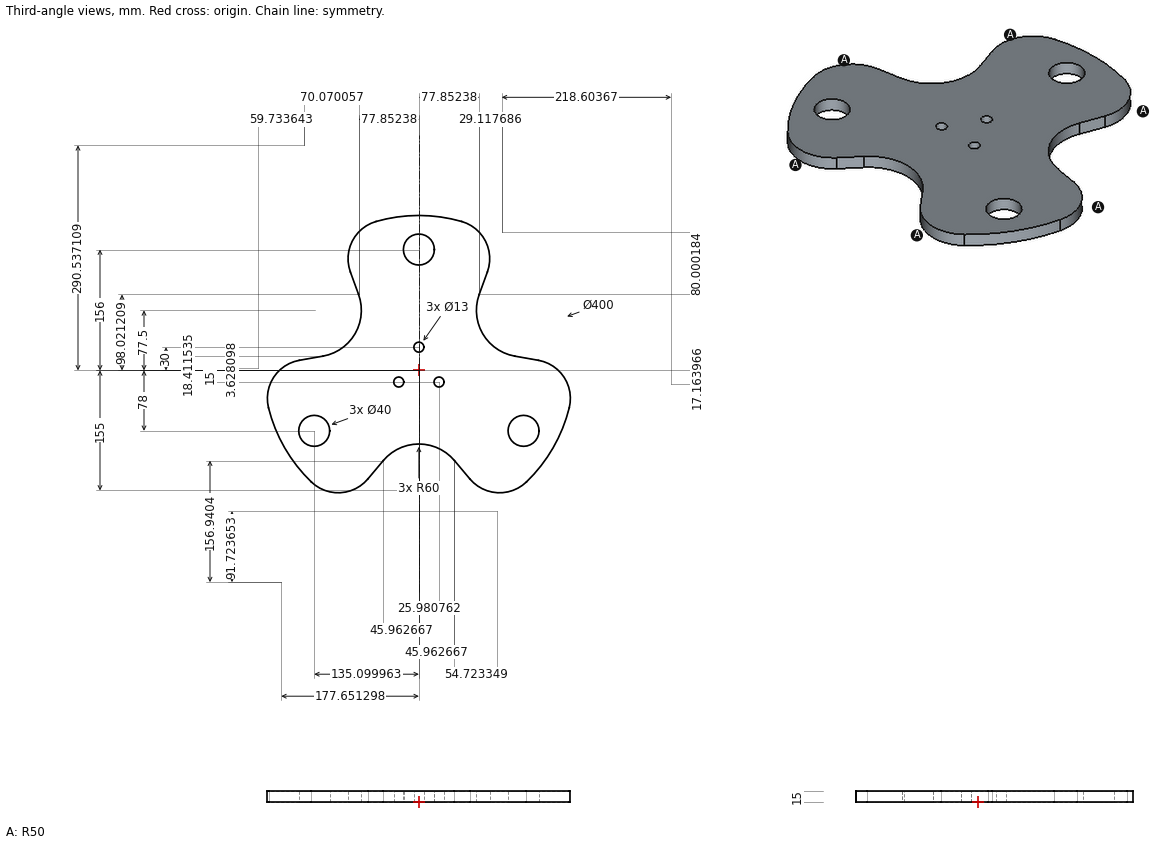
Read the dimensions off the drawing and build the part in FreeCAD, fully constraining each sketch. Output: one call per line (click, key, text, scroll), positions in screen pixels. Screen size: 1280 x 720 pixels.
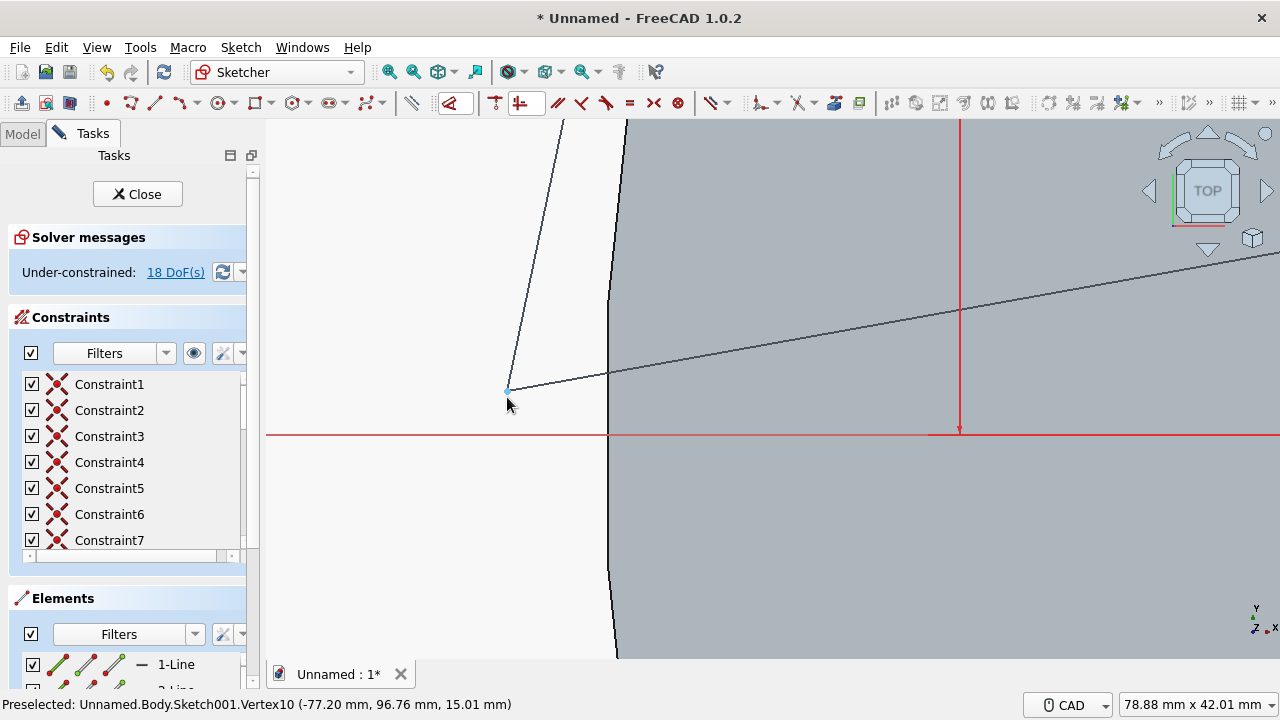
click(507, 391)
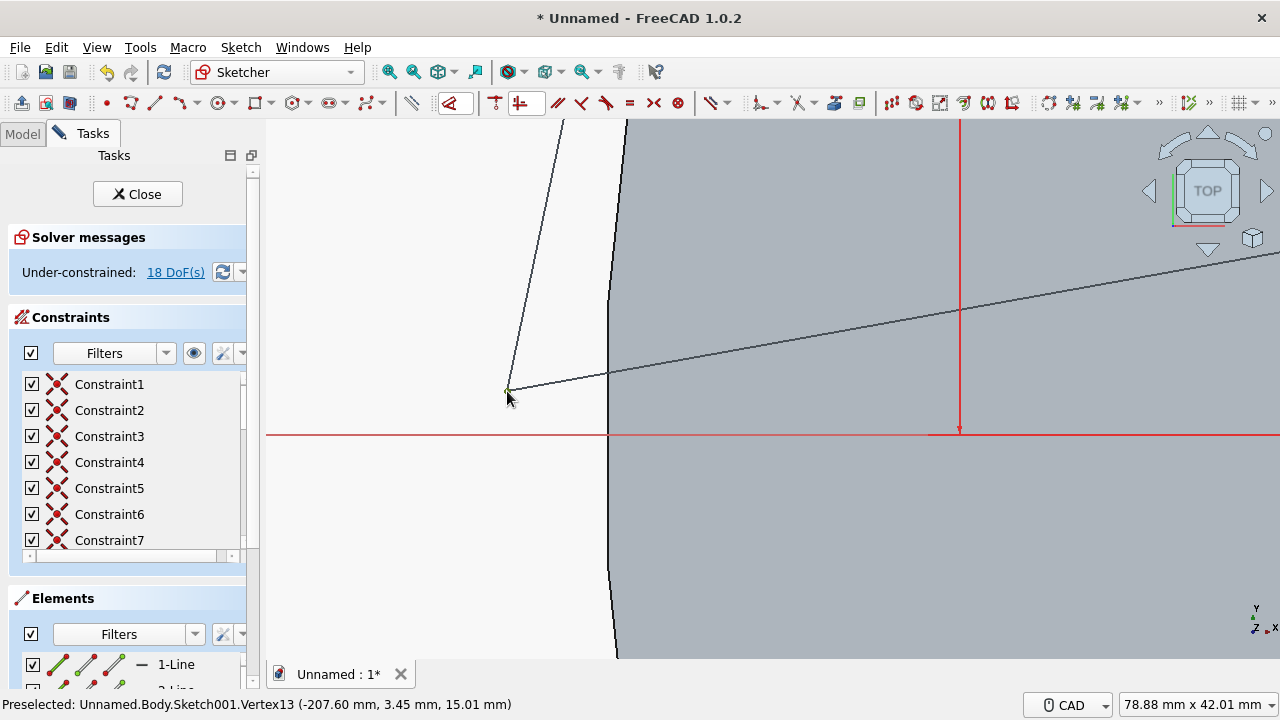
key(i)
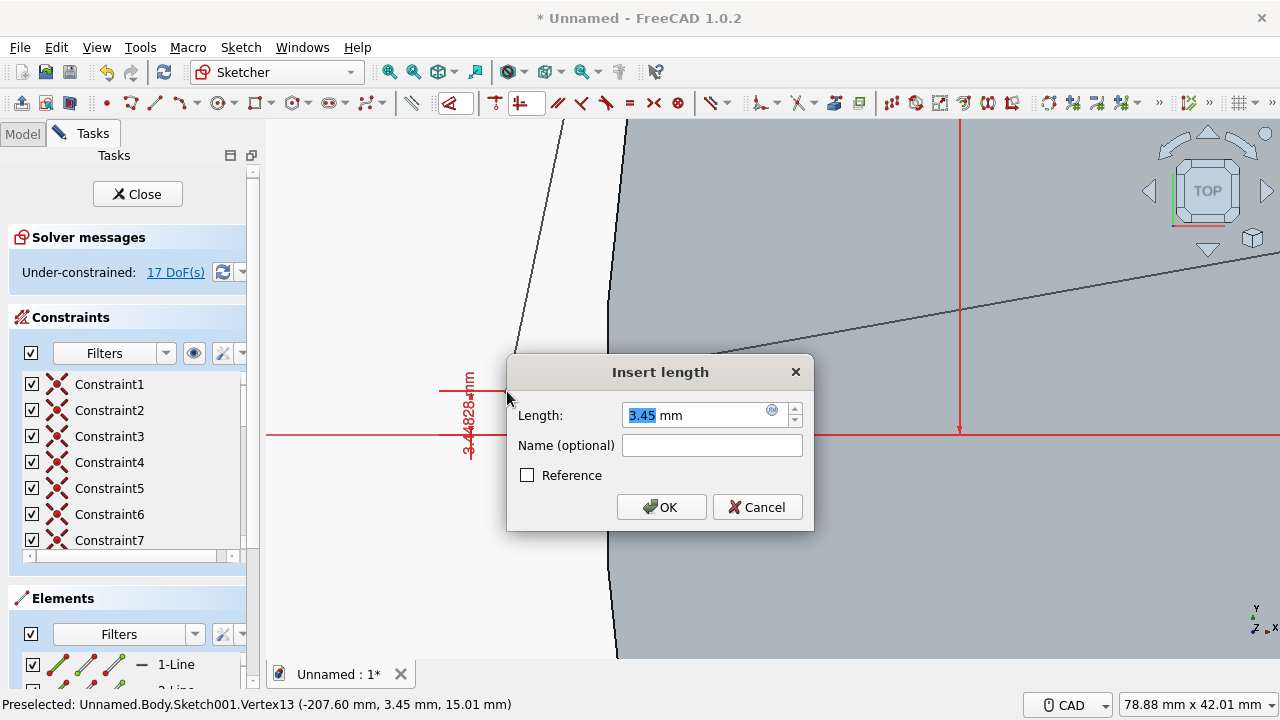
text(3.628098)
key(Return)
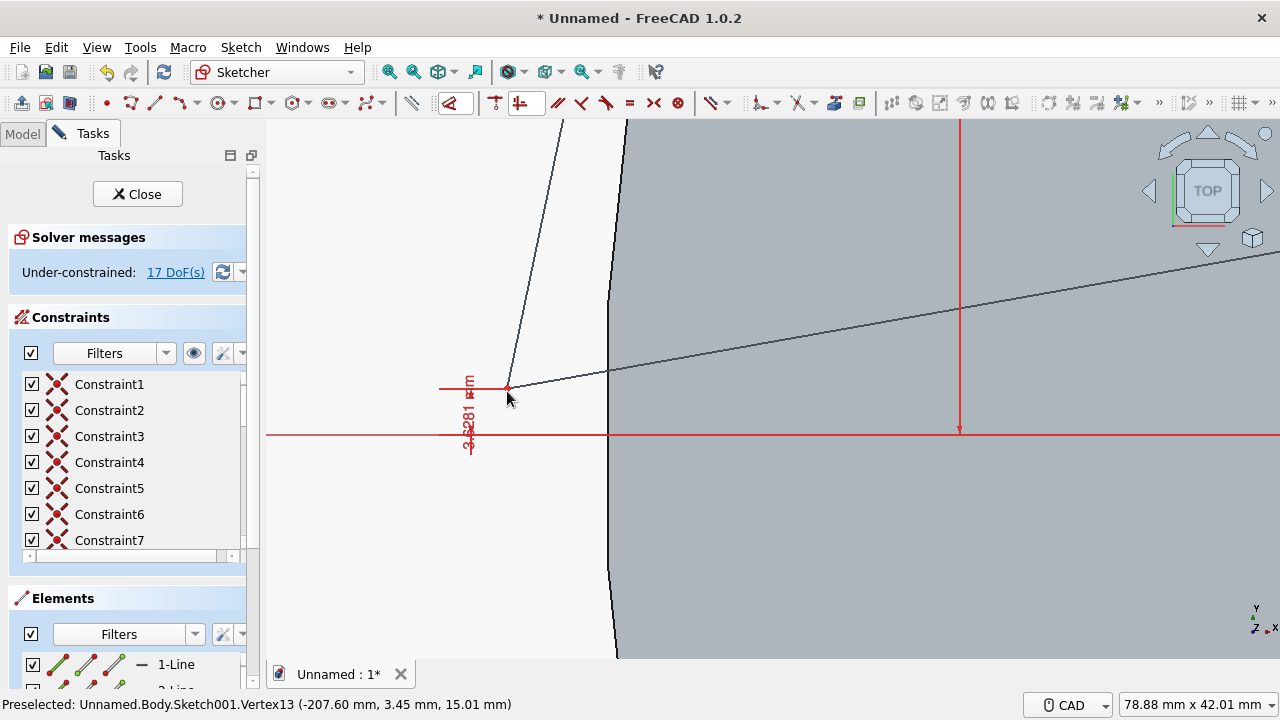
scroll(535, 392, down, 15)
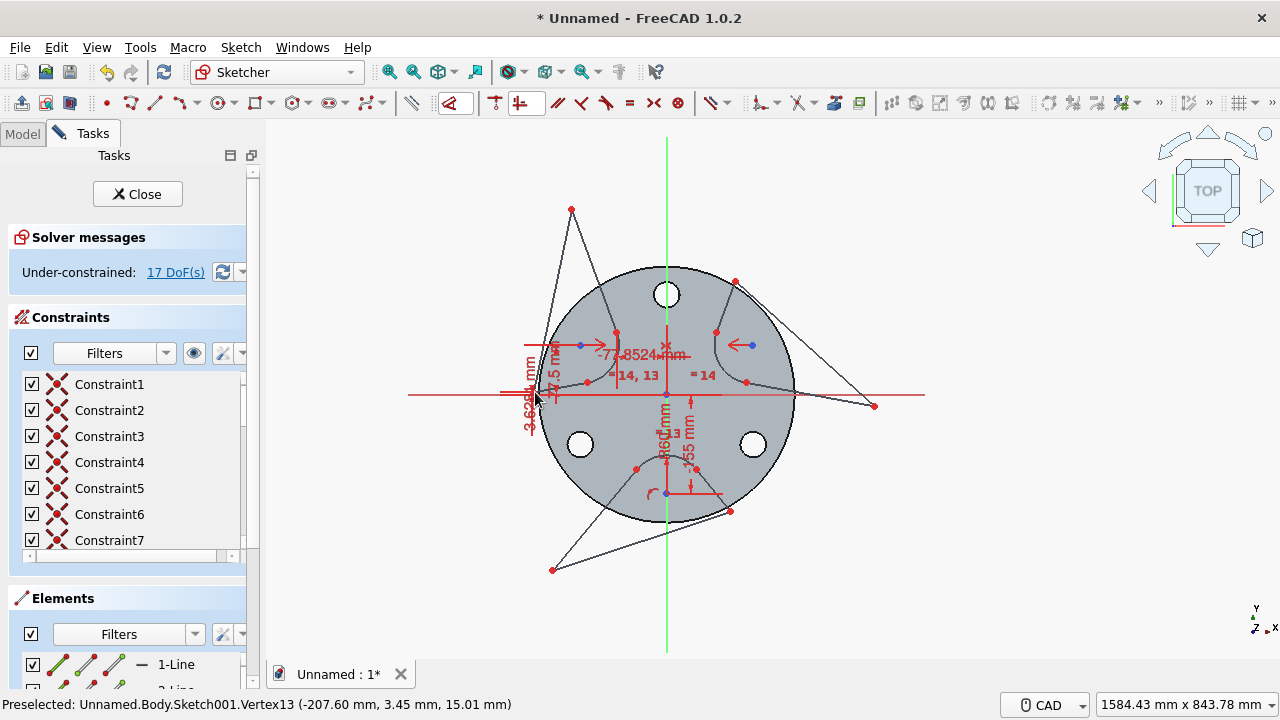
click(717, 333)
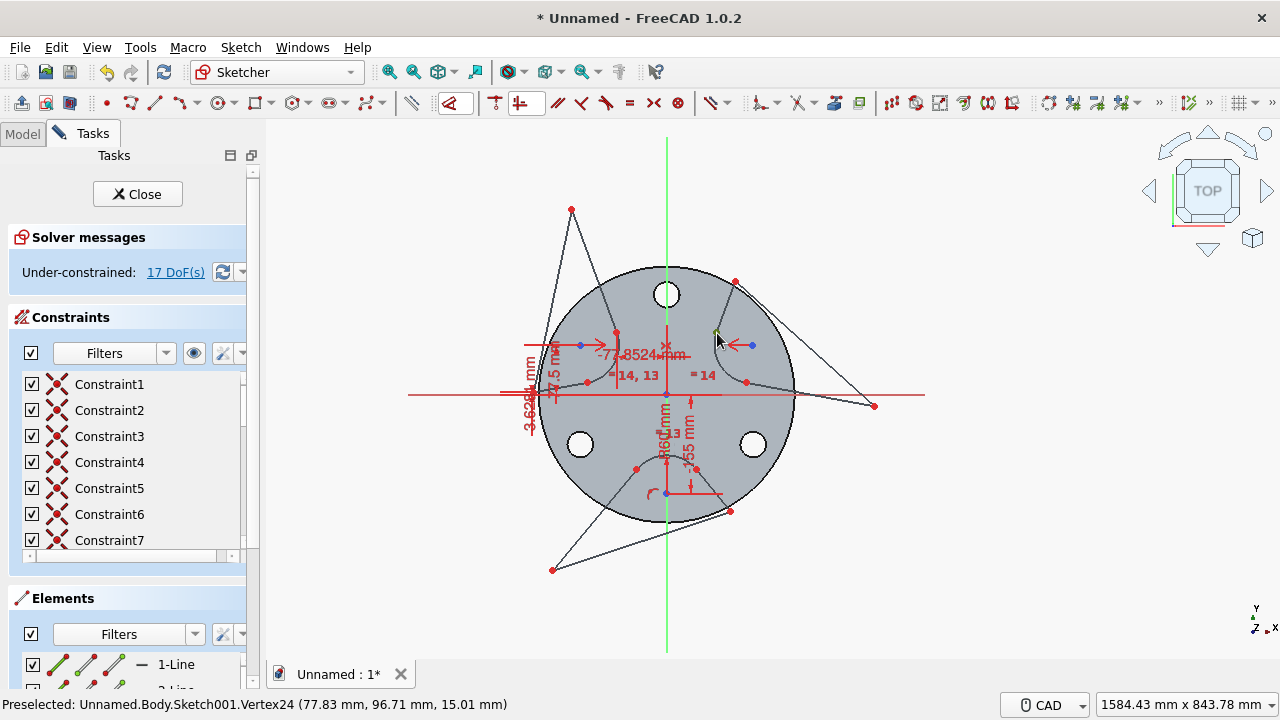
click(468, 104)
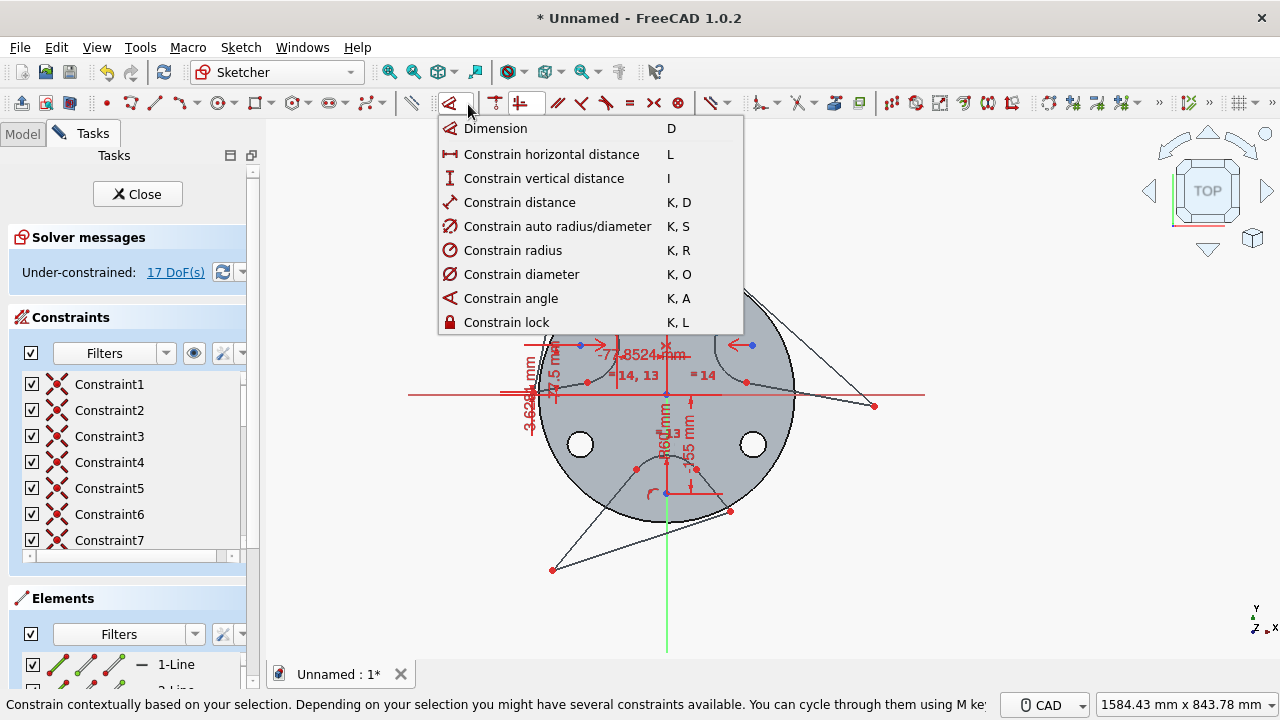
click(591, 154)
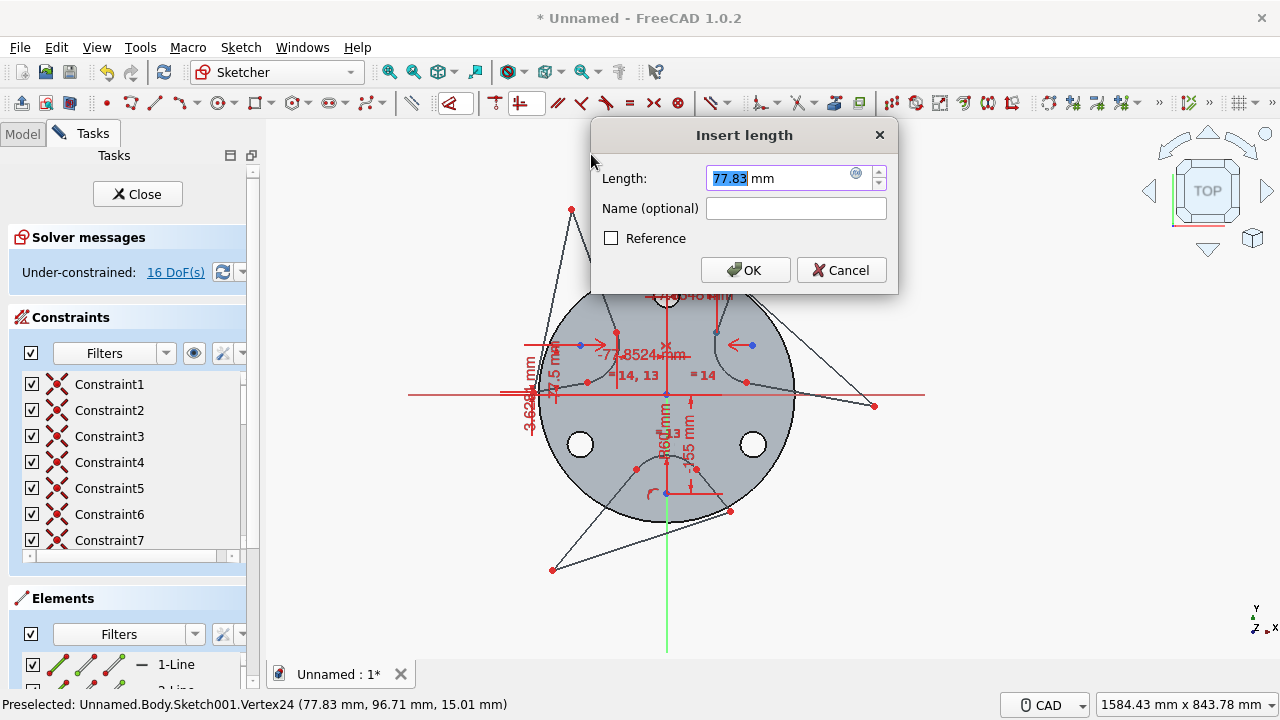
text(77.85238)
key(Return)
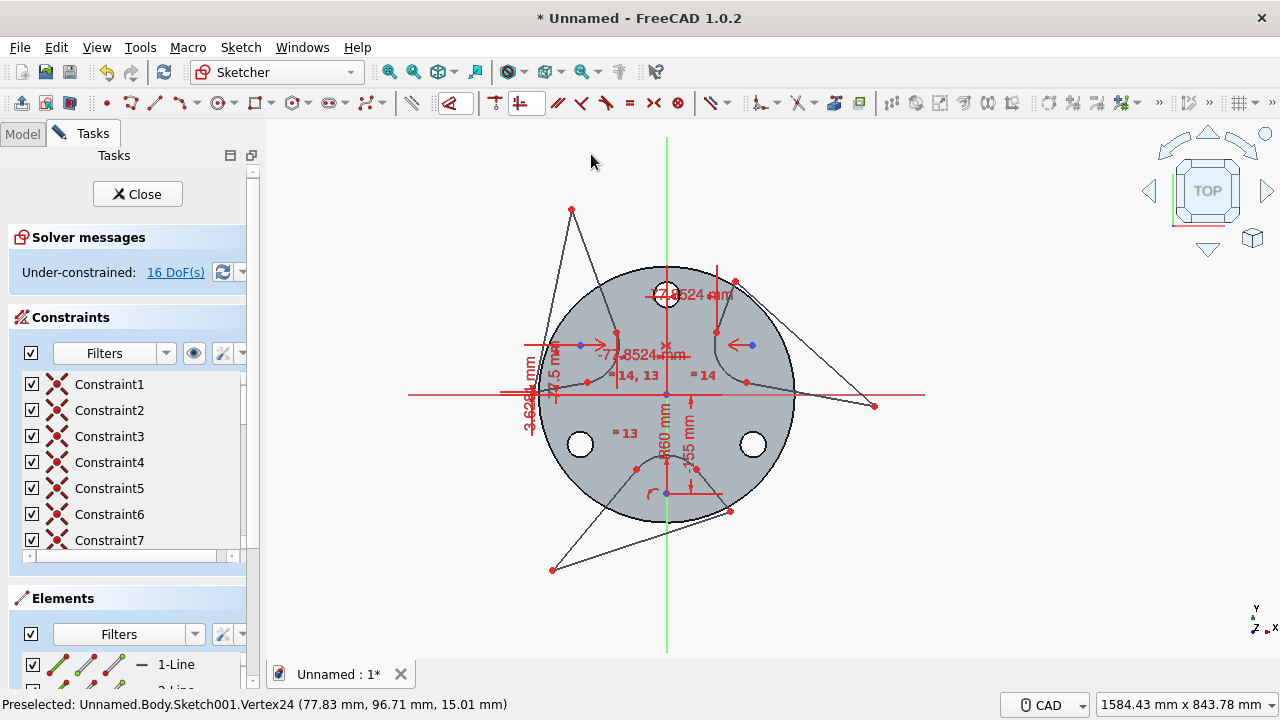
click(612, 500)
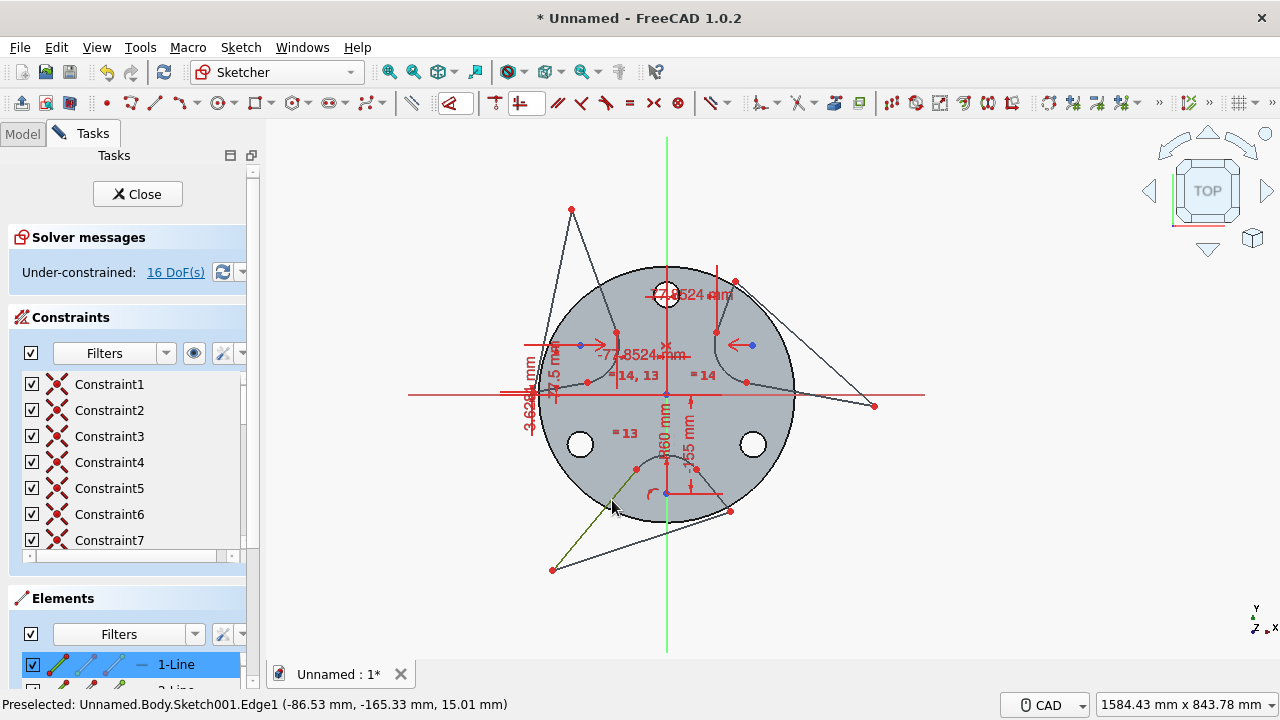
key(i)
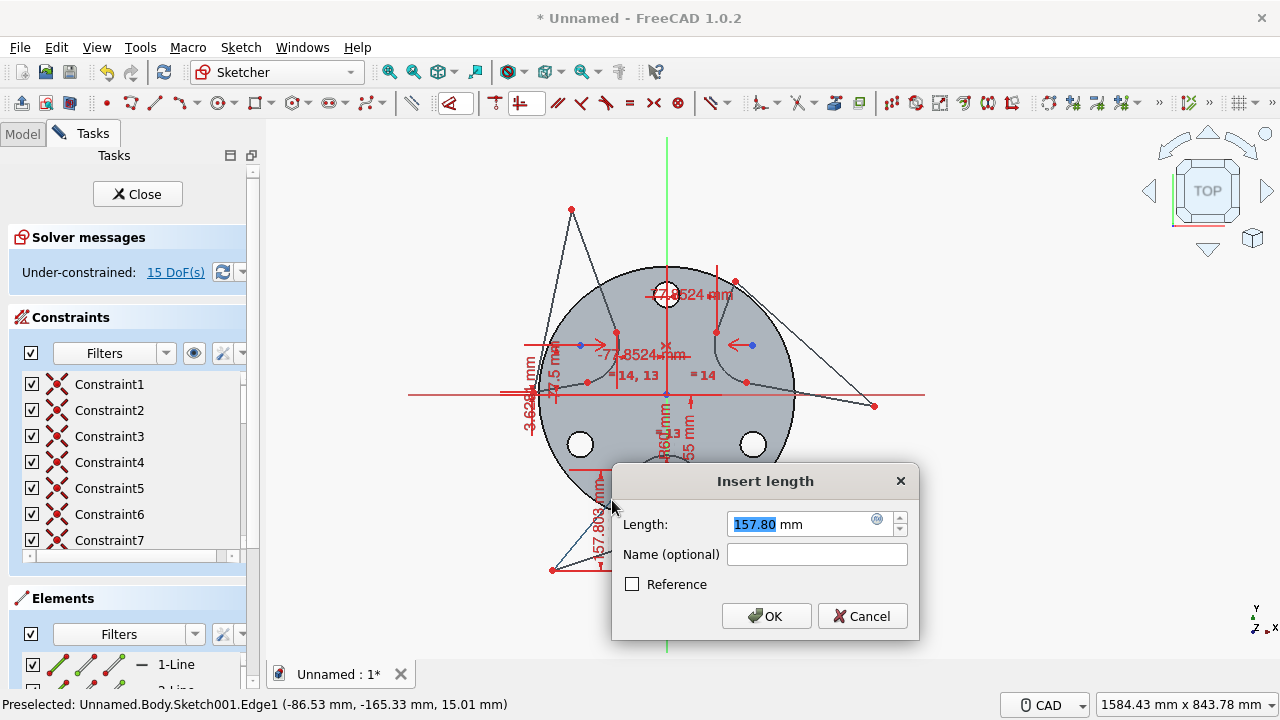
text(156.9404)
key(Return)